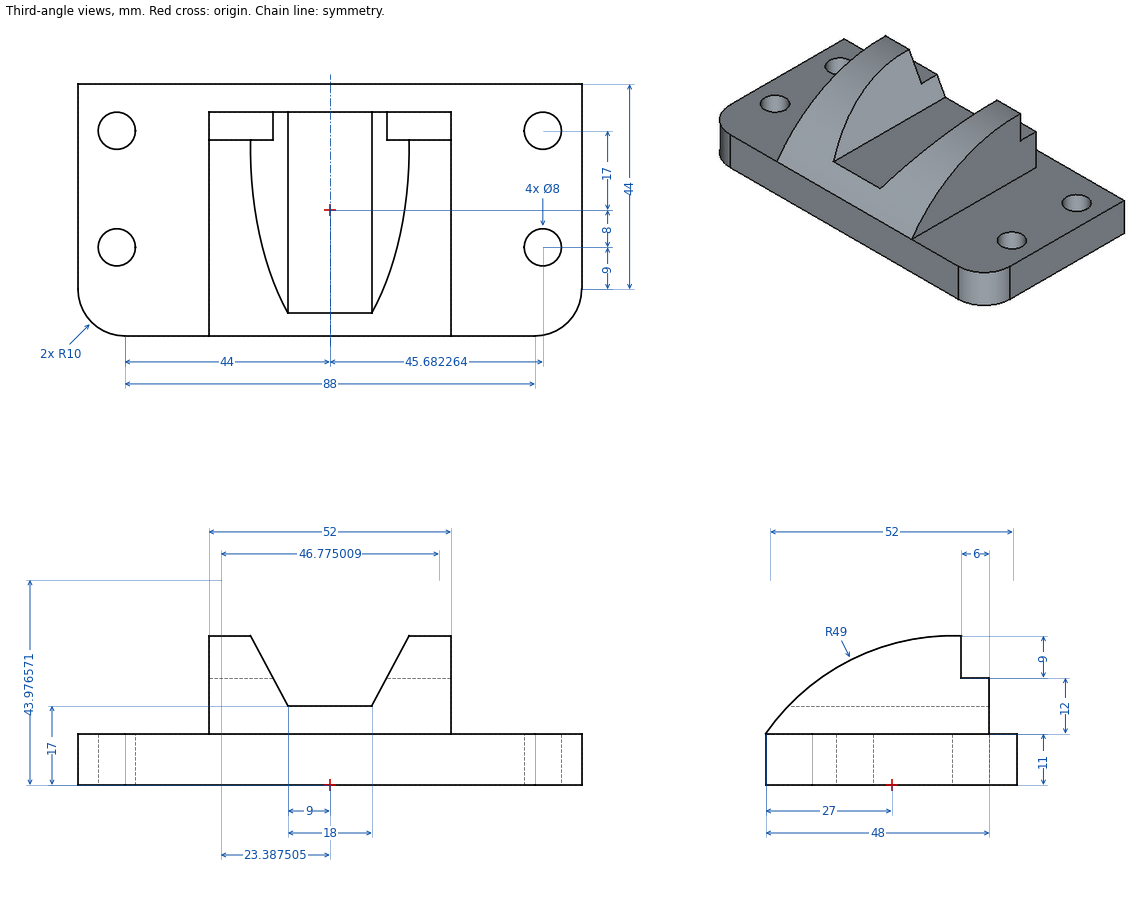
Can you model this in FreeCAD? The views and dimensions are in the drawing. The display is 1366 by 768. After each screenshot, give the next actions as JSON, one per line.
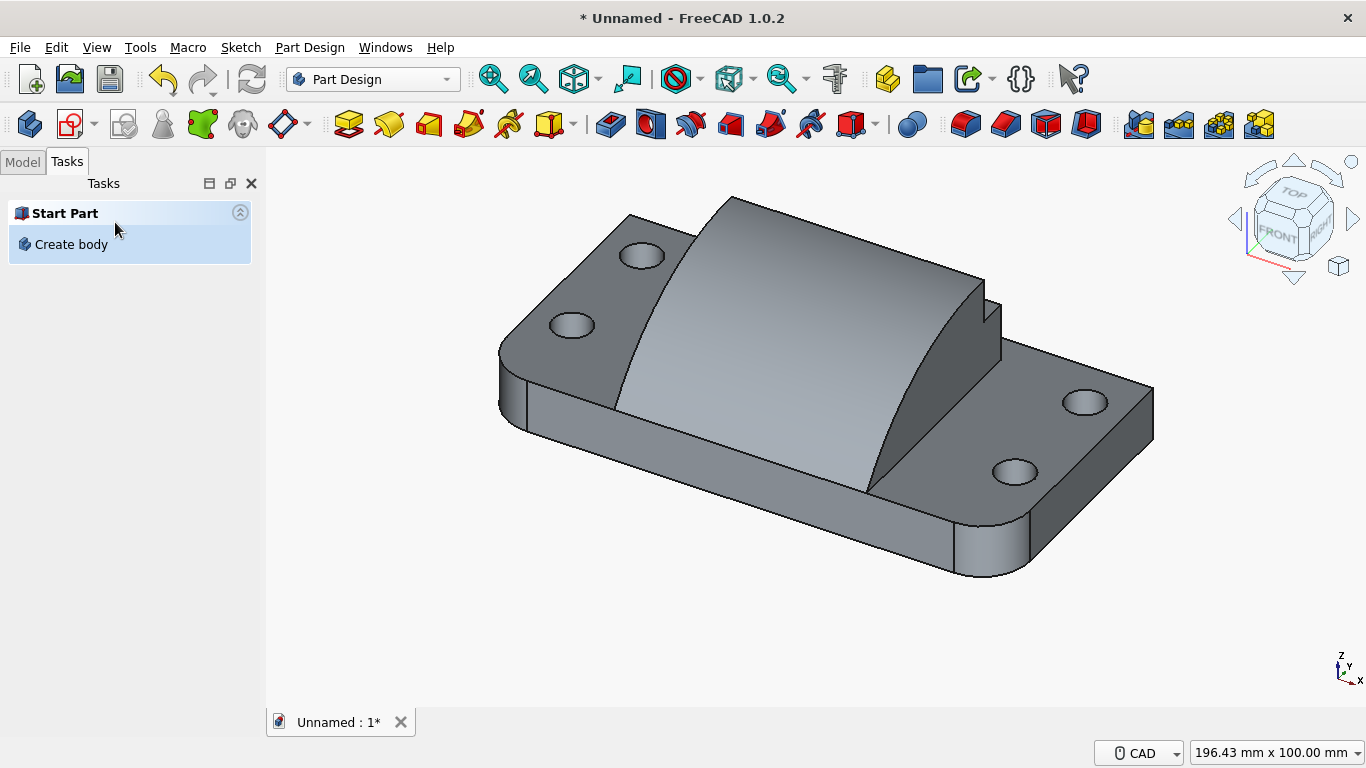
{"action": "left_click", "coordinate": [494, 80]}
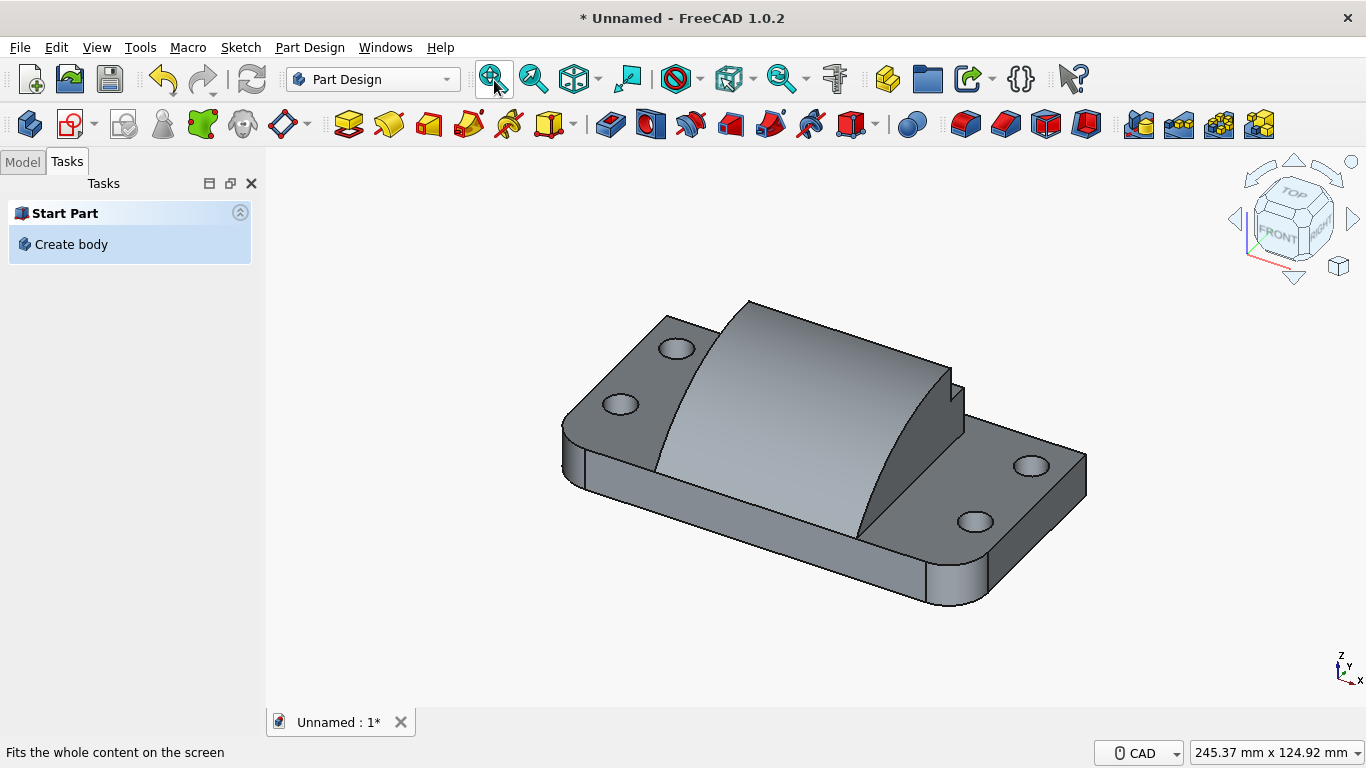
{"action": "left_click", "coordinate": [70, 124]}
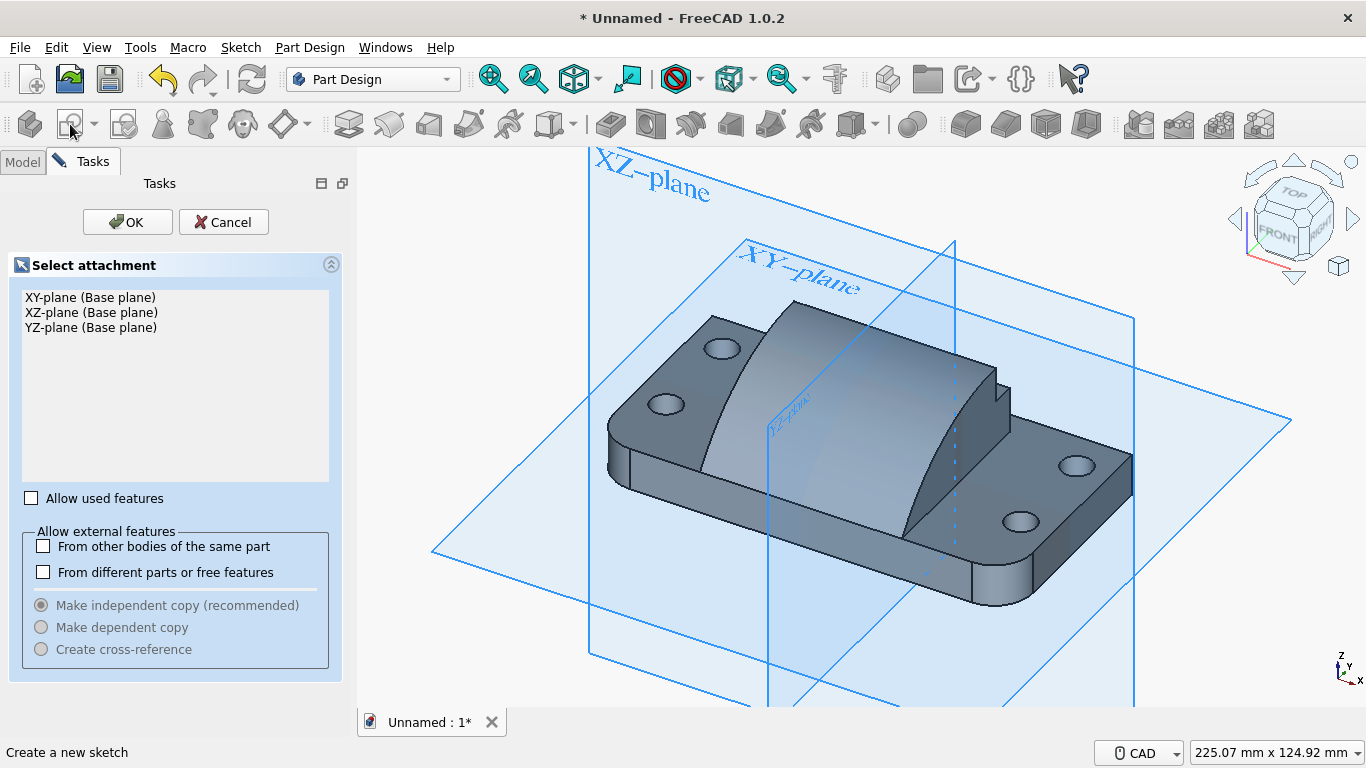
{"action": "left_click", "coordinate": [82, 312]}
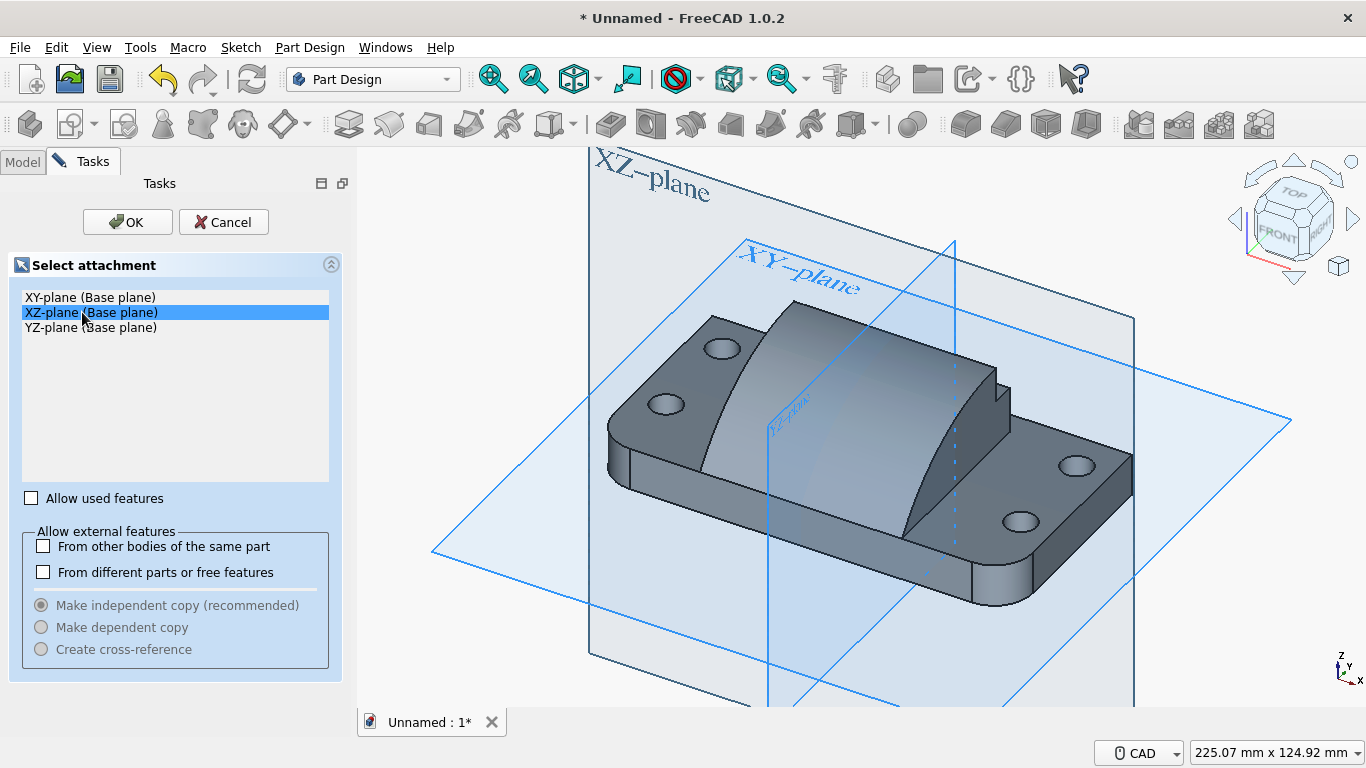
{"action": "left_click", "coordinate": [128, 222]}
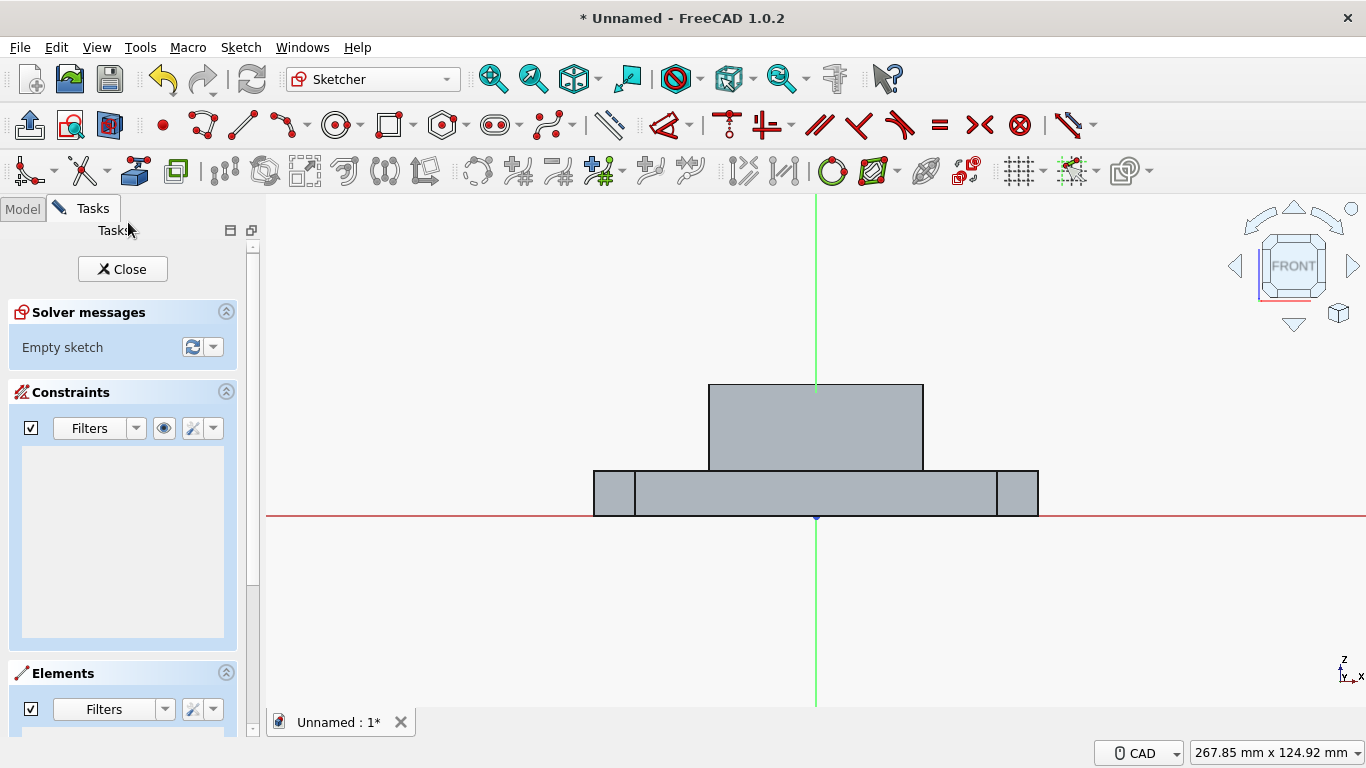
{"action": "left_click", "coordinate": [110, 126]}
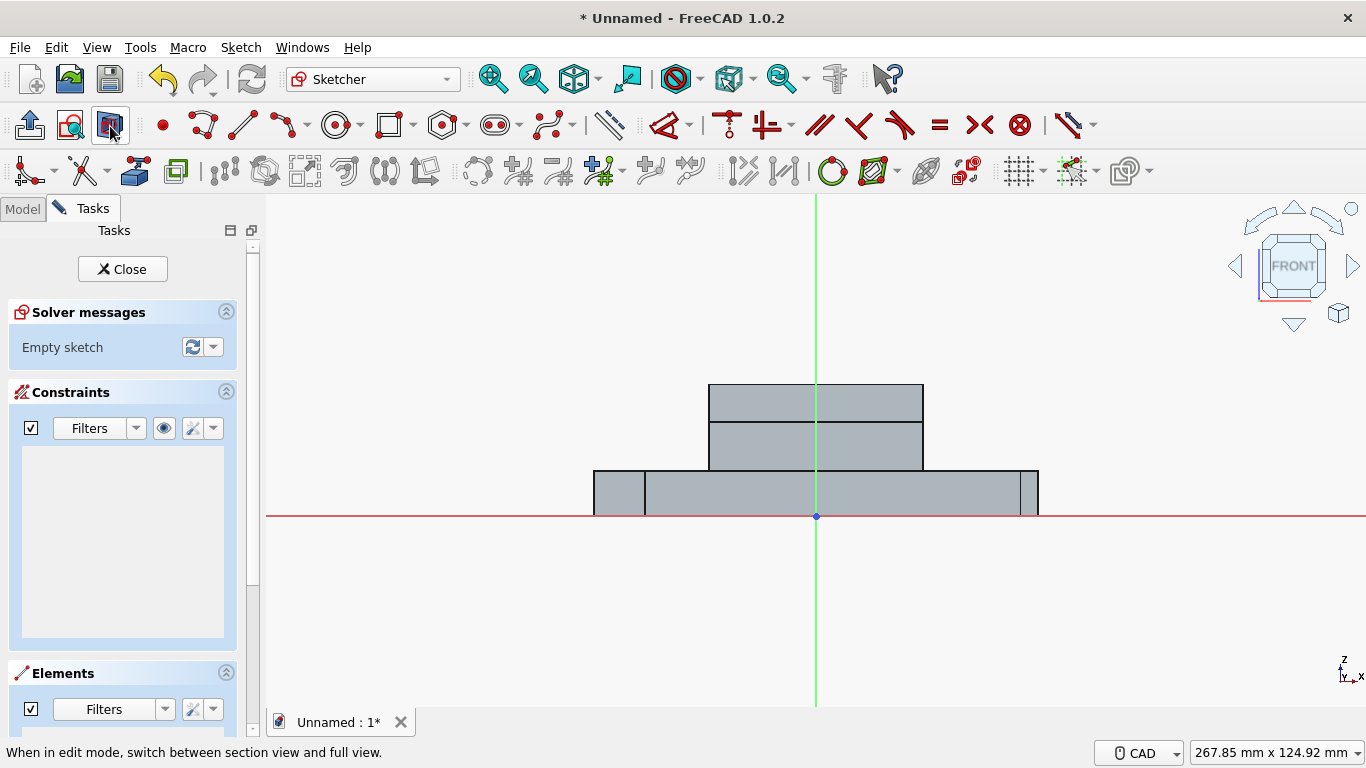
{"action": "scroll", "coordinate": [899, 396], "scroll_direction": "up", "scroll_amount": 3}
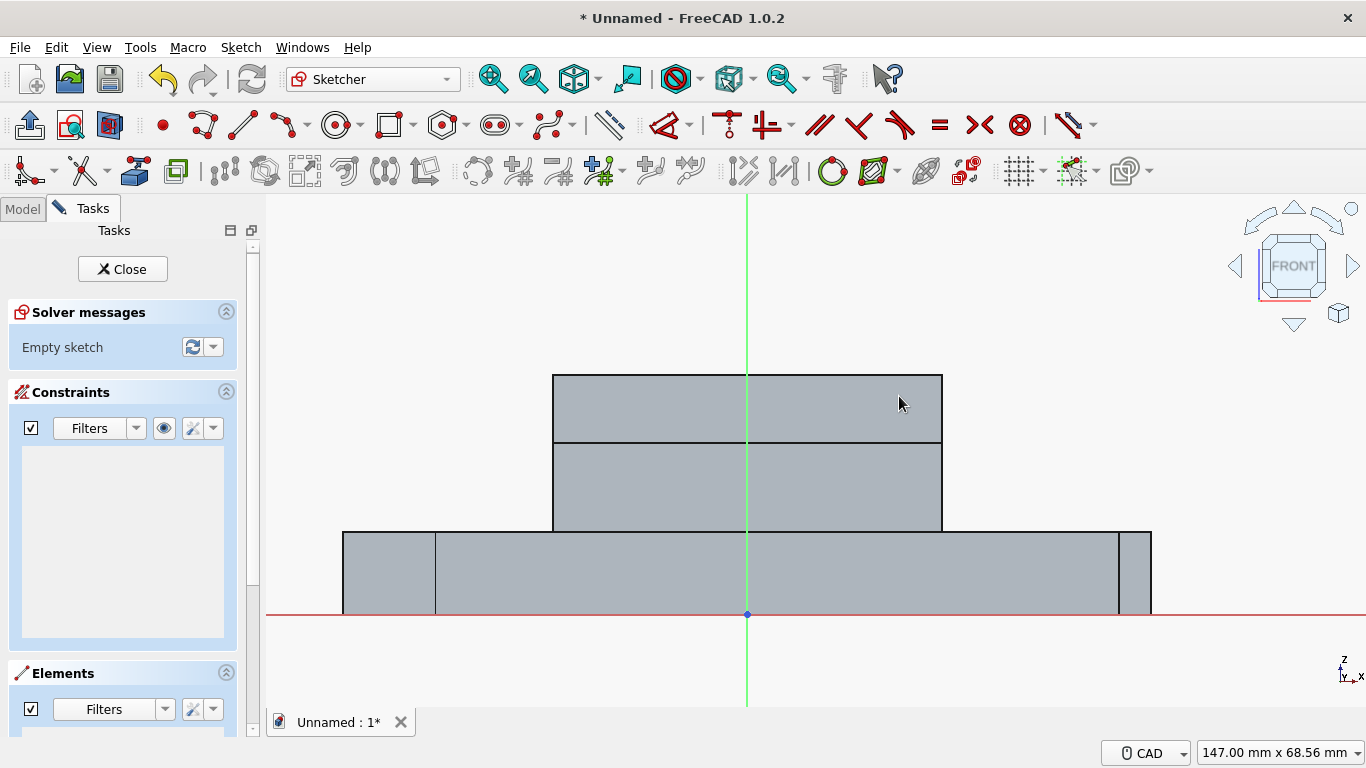
{"action": "left_click", "coordinate": [204, 126]}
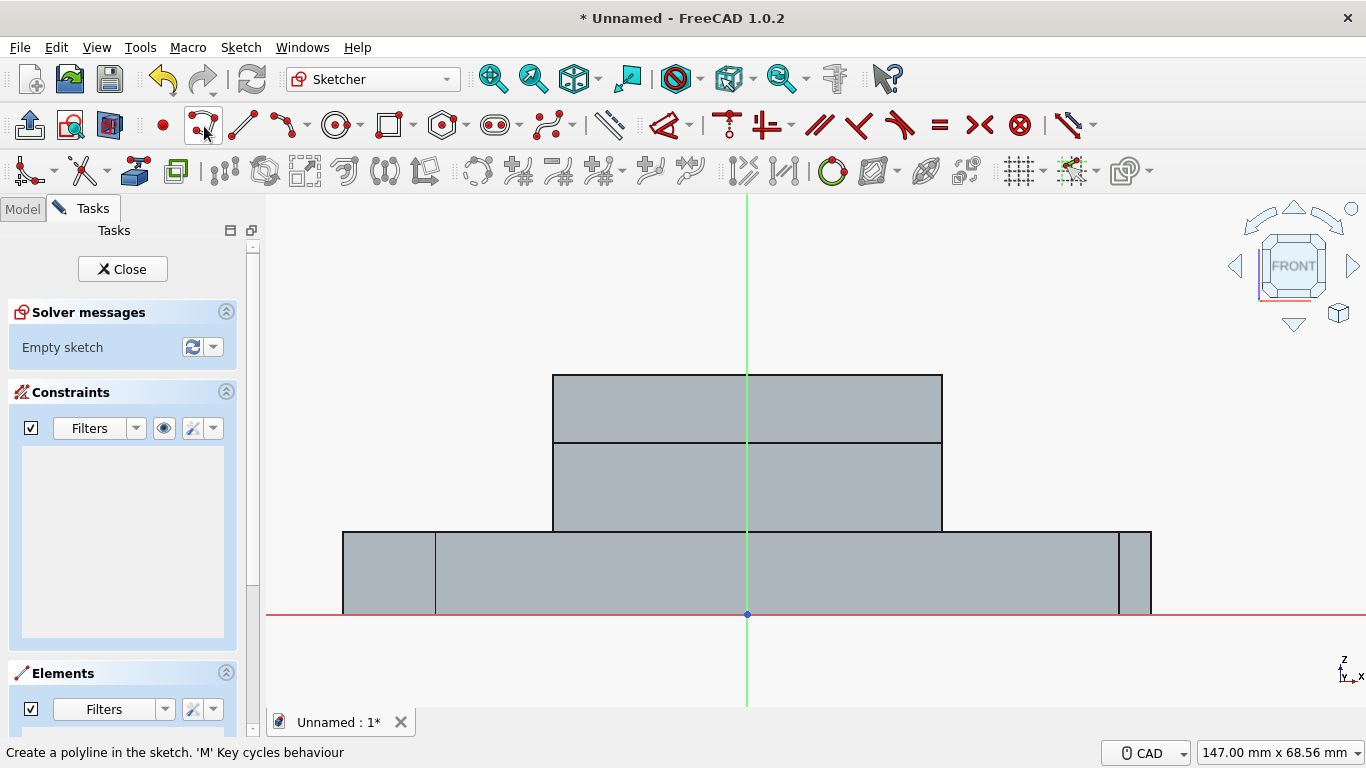
{"action": "left_click", "coordinate": [680, 487]}
{"action": "left_click", "coordinate": [572, 286]}
{"action": "left_click", "coordinate": [922, 286]}
{"action": "left_click", "coordinate": [815, 487]}
{"action": "left_click", "coordinate": [680, 488]}
{"action": "key", "text": "Escape"}
{"action": "key", "text": "Escape"}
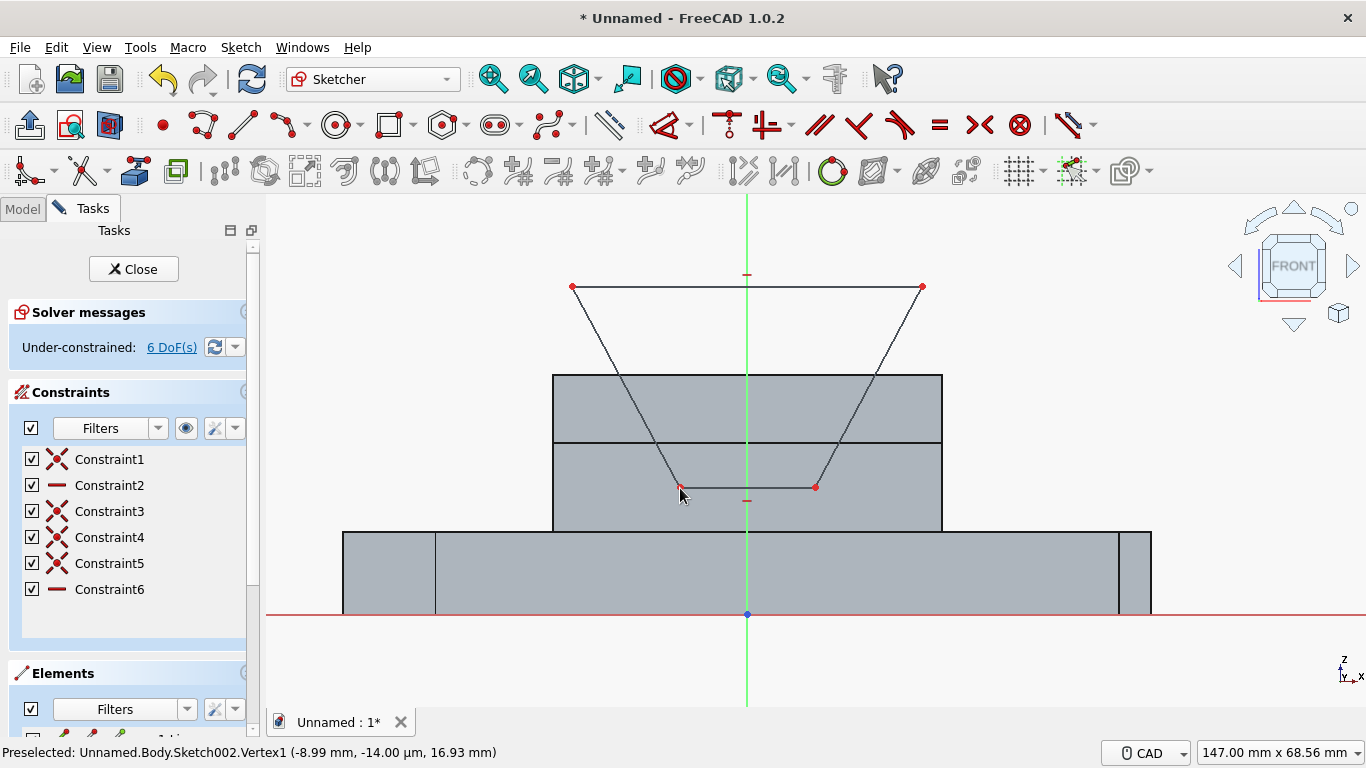
{"action": "left_click", "coordinate": [664, 126]}